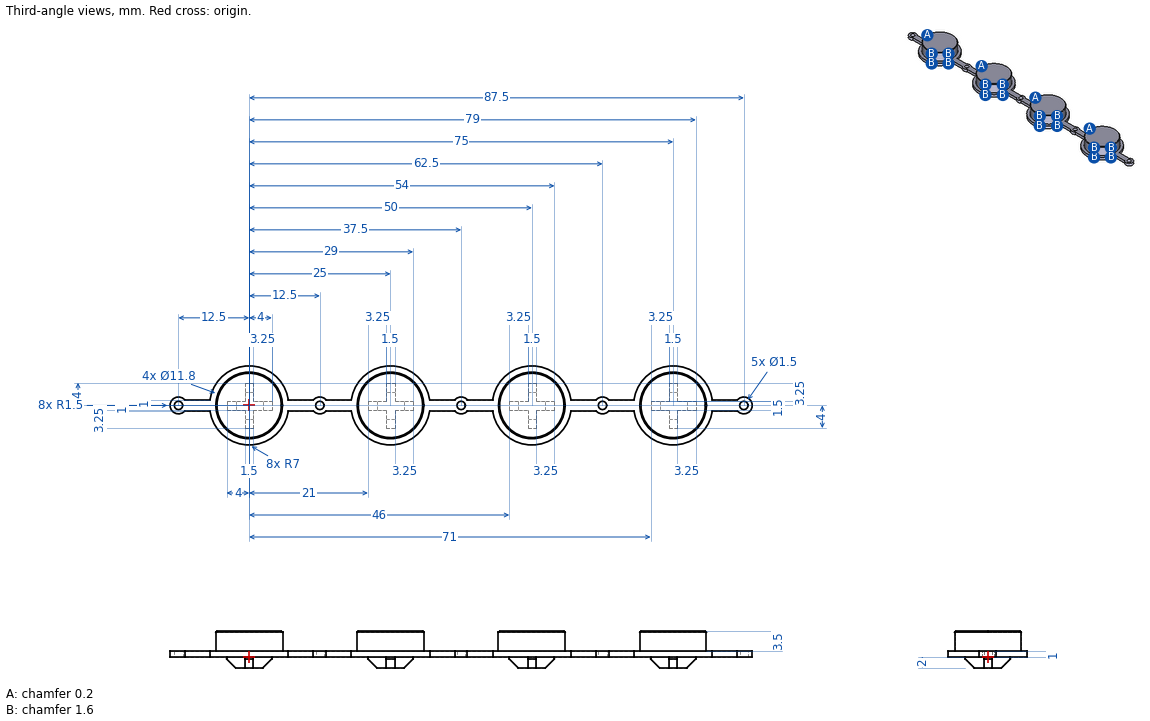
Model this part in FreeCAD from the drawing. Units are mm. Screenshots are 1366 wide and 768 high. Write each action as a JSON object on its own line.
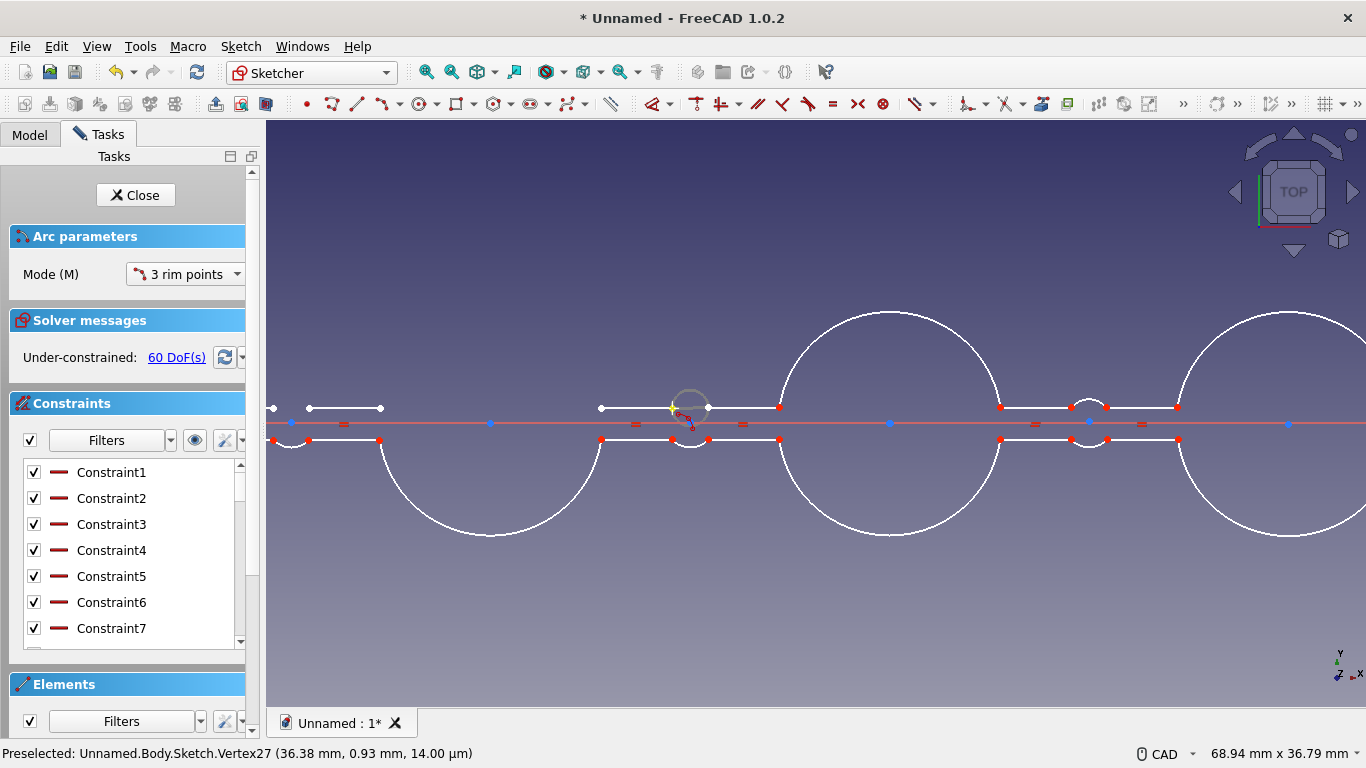
{"action": "scroll", "coordinate": [690, 399], "scroll_direction": "up", "scroll_amount": 4}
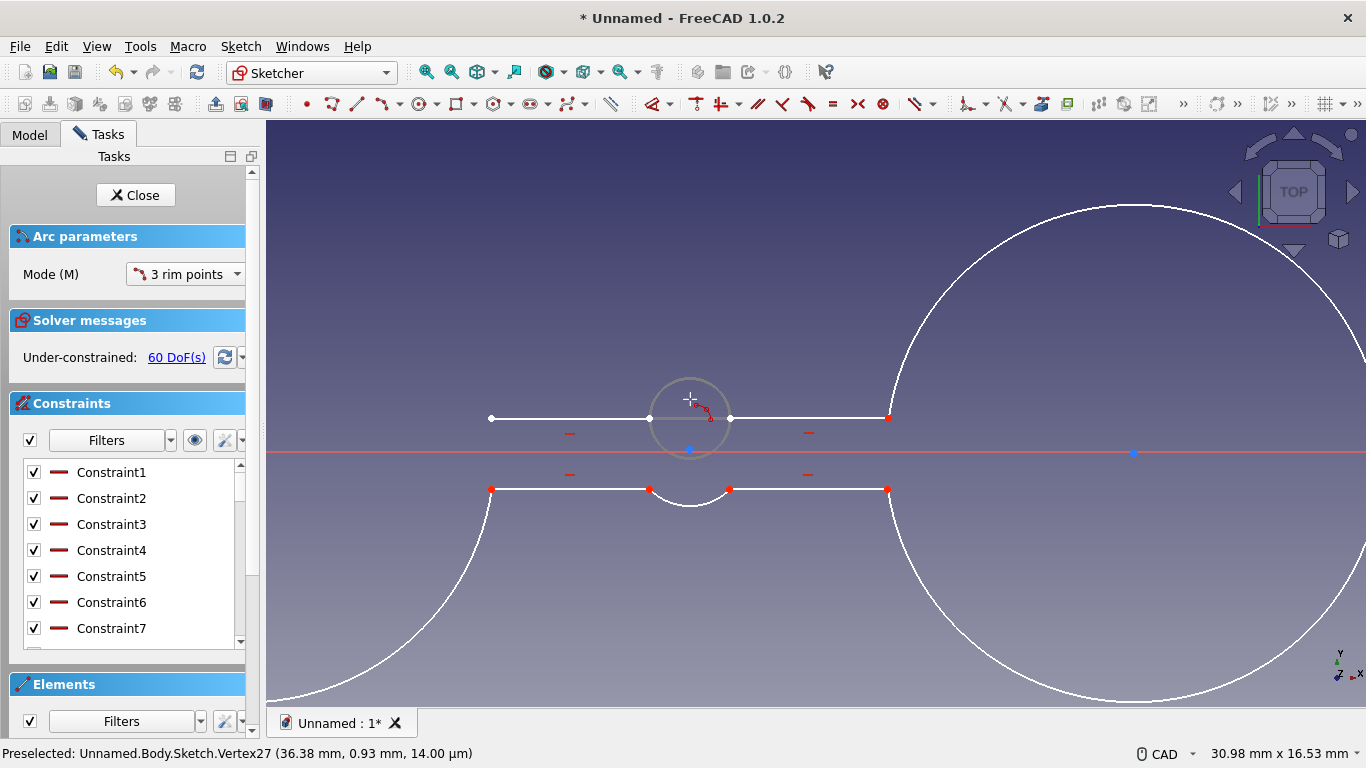
{"action": "left_click", "coordinate": [690, 399]}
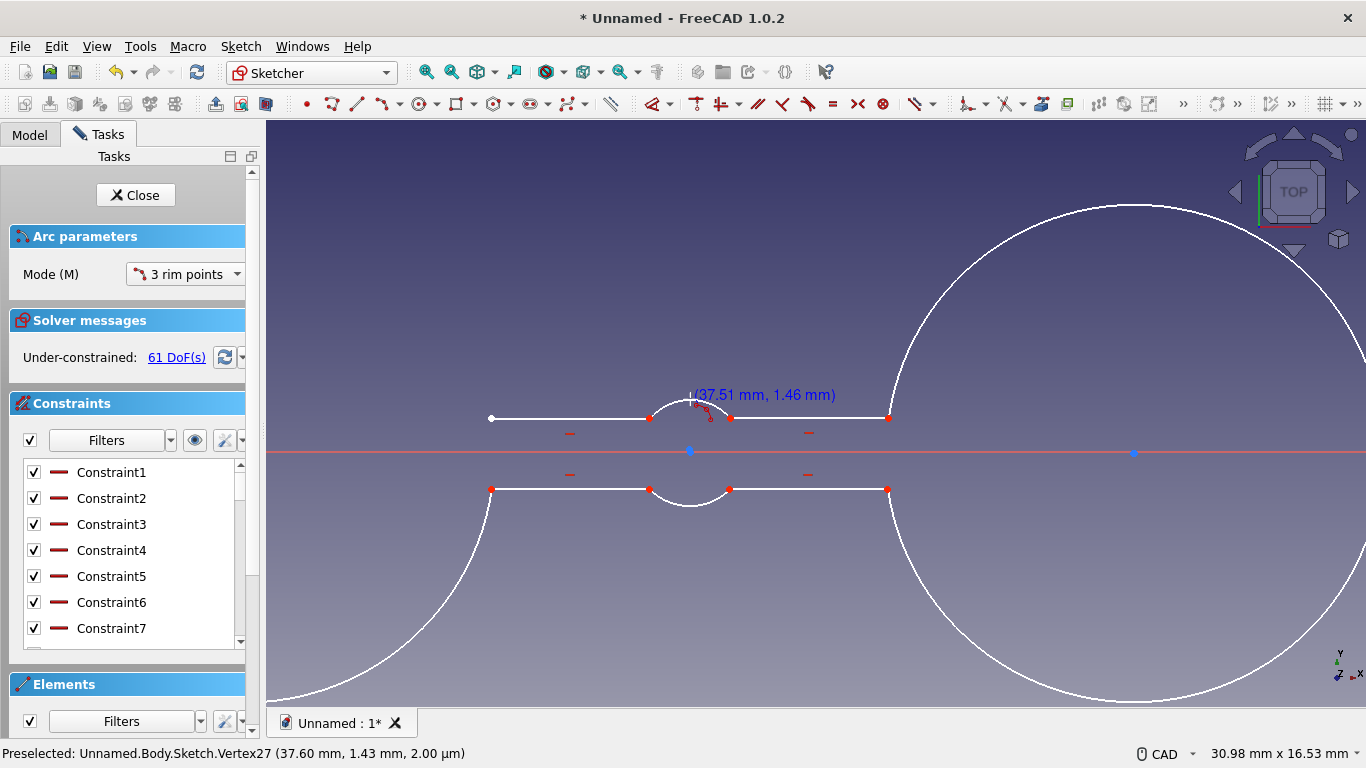
{"action": "left_click", "coordinate": [492, 419]}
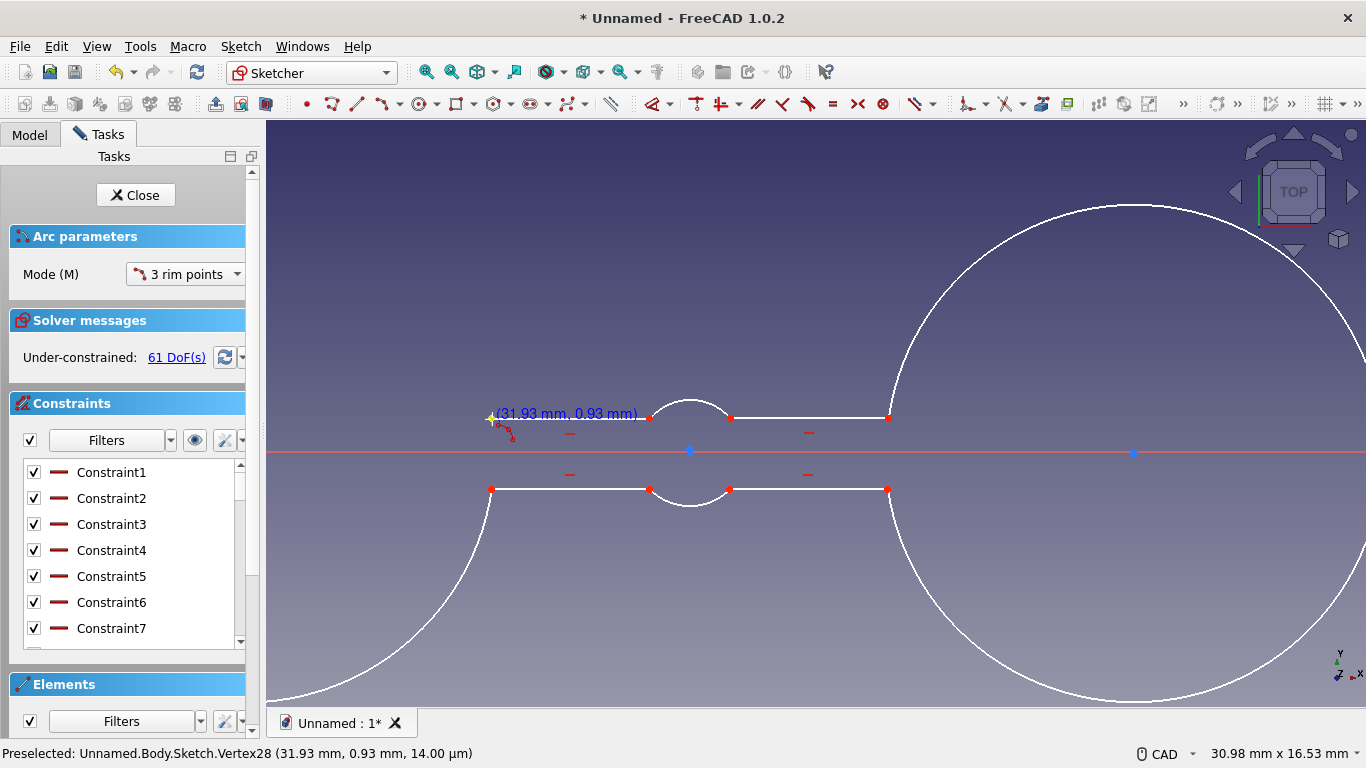
{"action": "scroll", "coordinate": [759, 406], "scroll_direction": "down", "scroll_amount": 9}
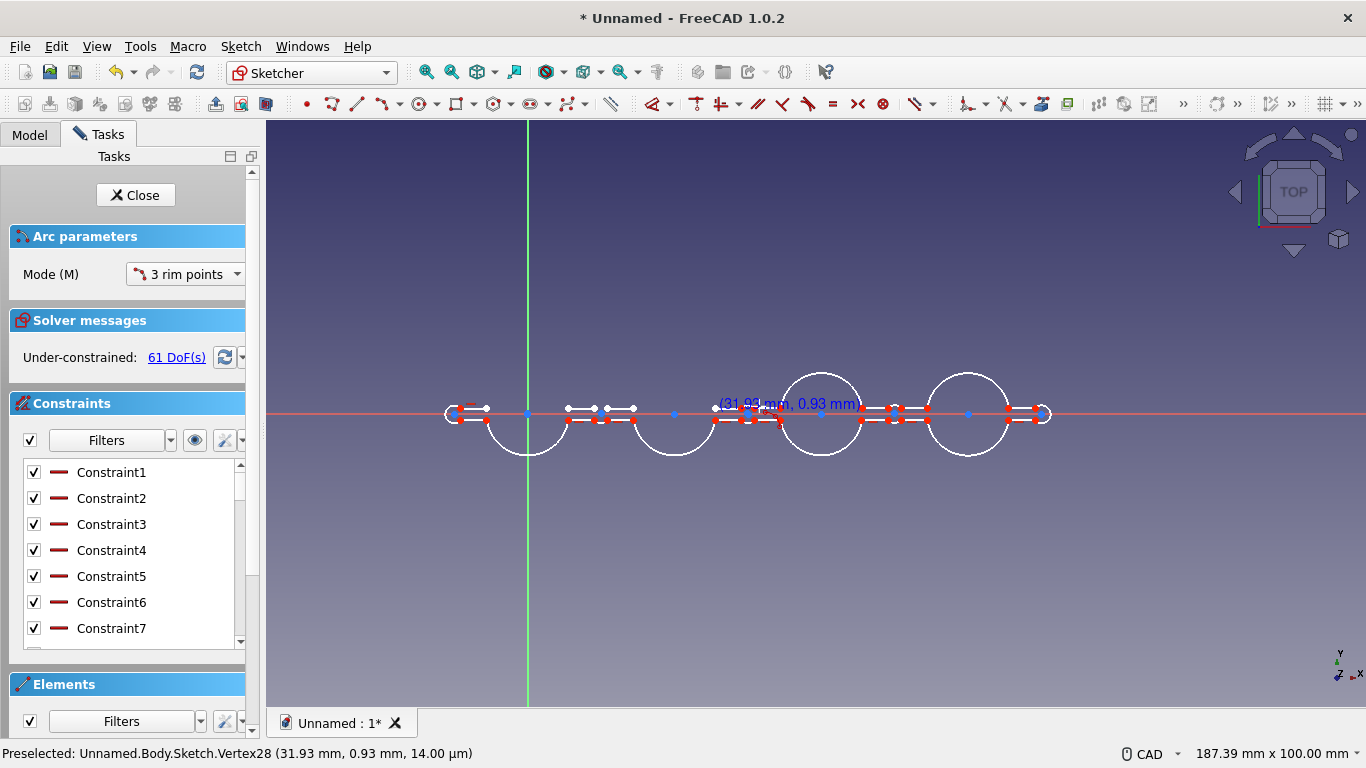
{"action": "scroll", "coordinate": [634, 408], "scroll_direction": "up", "scroll_amount": 5}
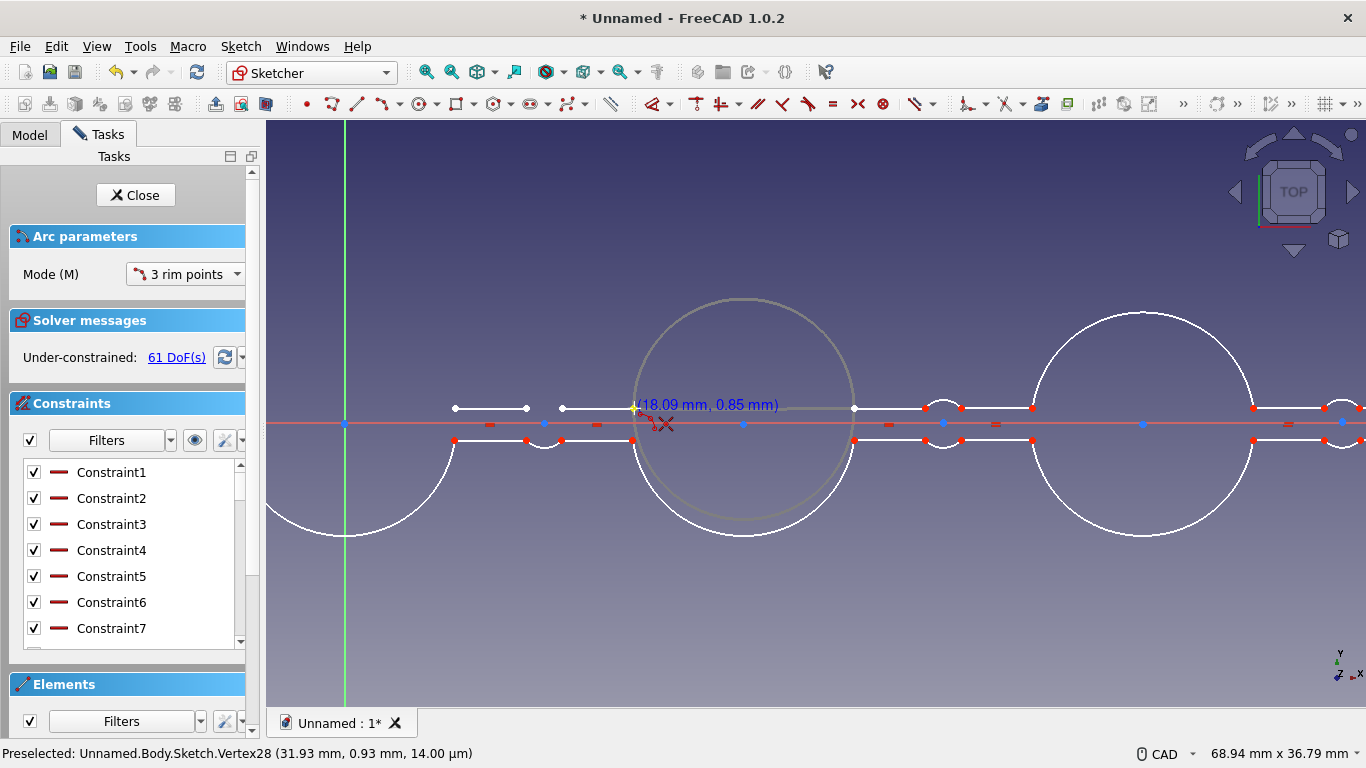
{"action": "left_click", "coordinate": [633, 409]}
{"action": "left_click", "coordinate": [744, 312]}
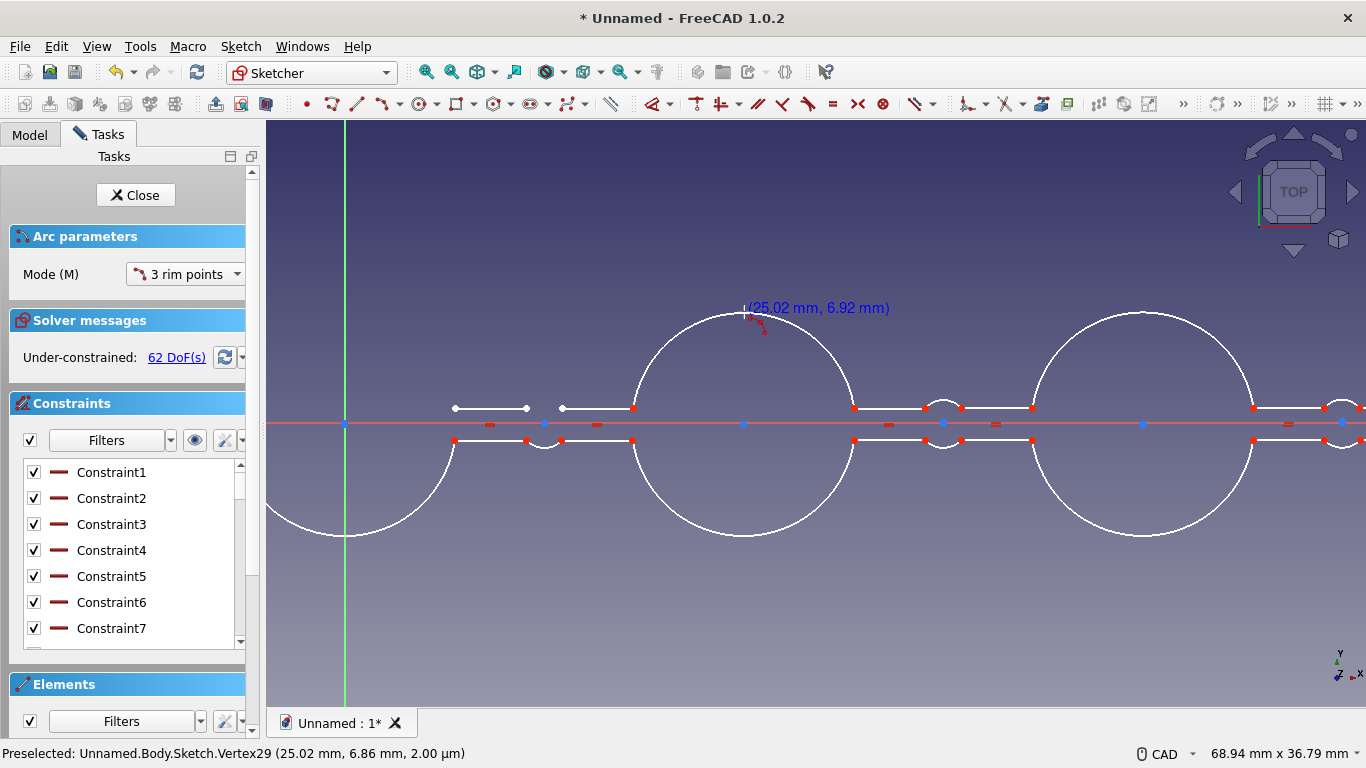
{"action": "left_click", "coordinate": [562, 409]}
{"action": "left_click", "coordinate": [526, 409]}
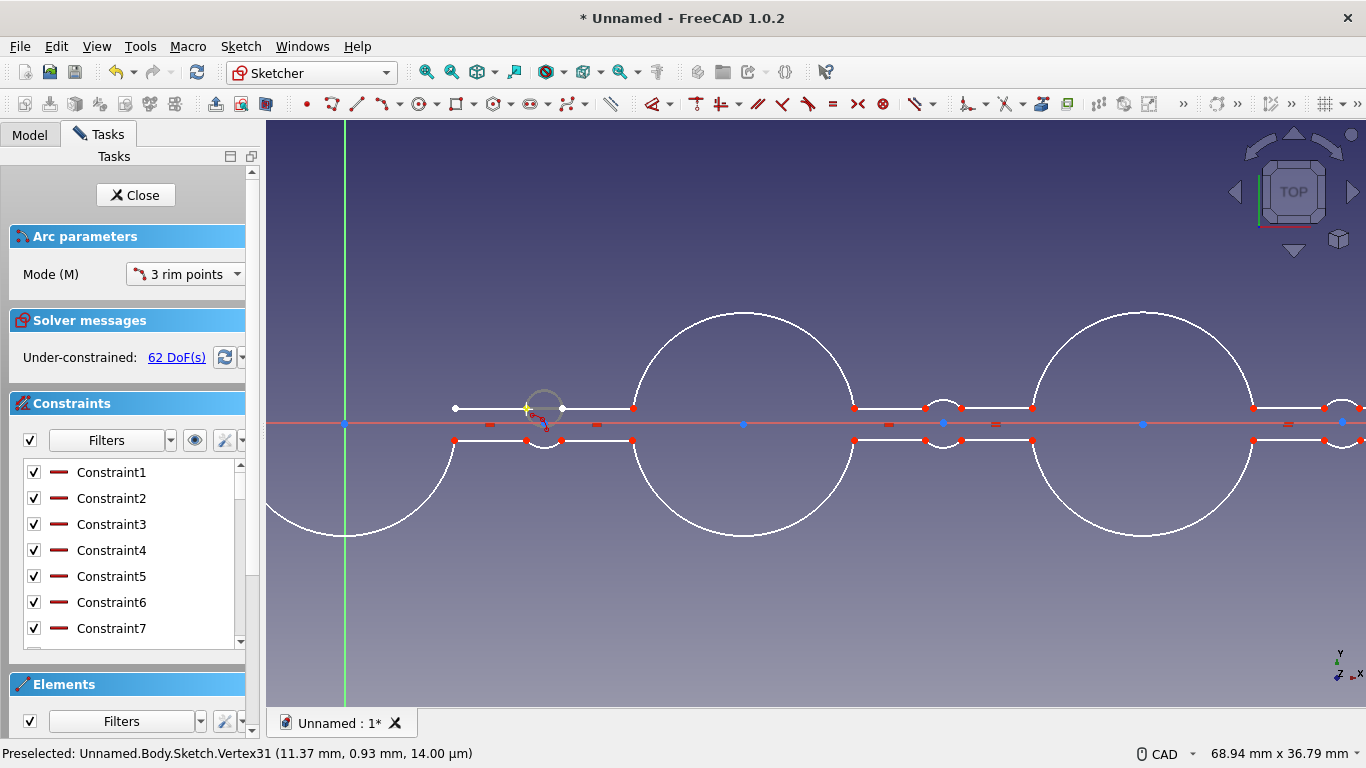
{"action": "scroll", "coordinate": [544, 399], "scroll_direction": "up", "scroll_amount": 4}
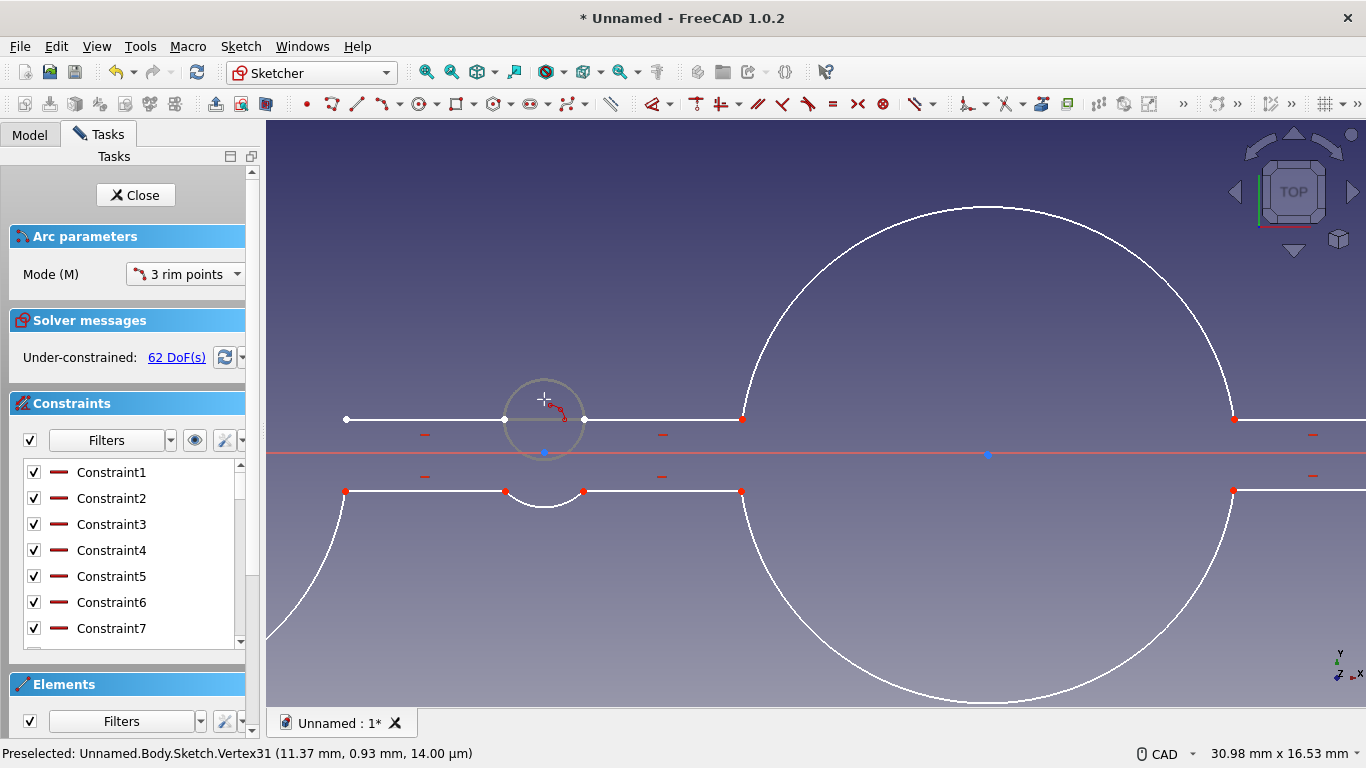
{"action": "left_click", "coordinate": [544, 399]}